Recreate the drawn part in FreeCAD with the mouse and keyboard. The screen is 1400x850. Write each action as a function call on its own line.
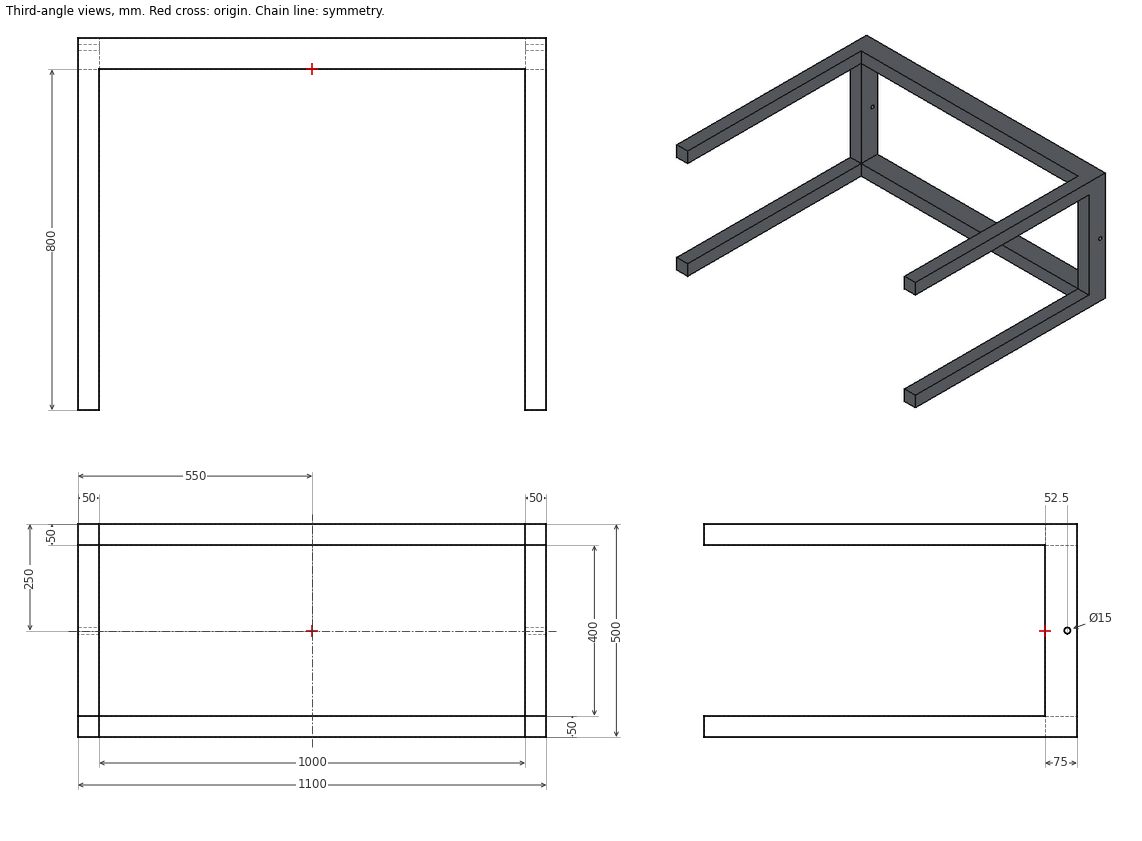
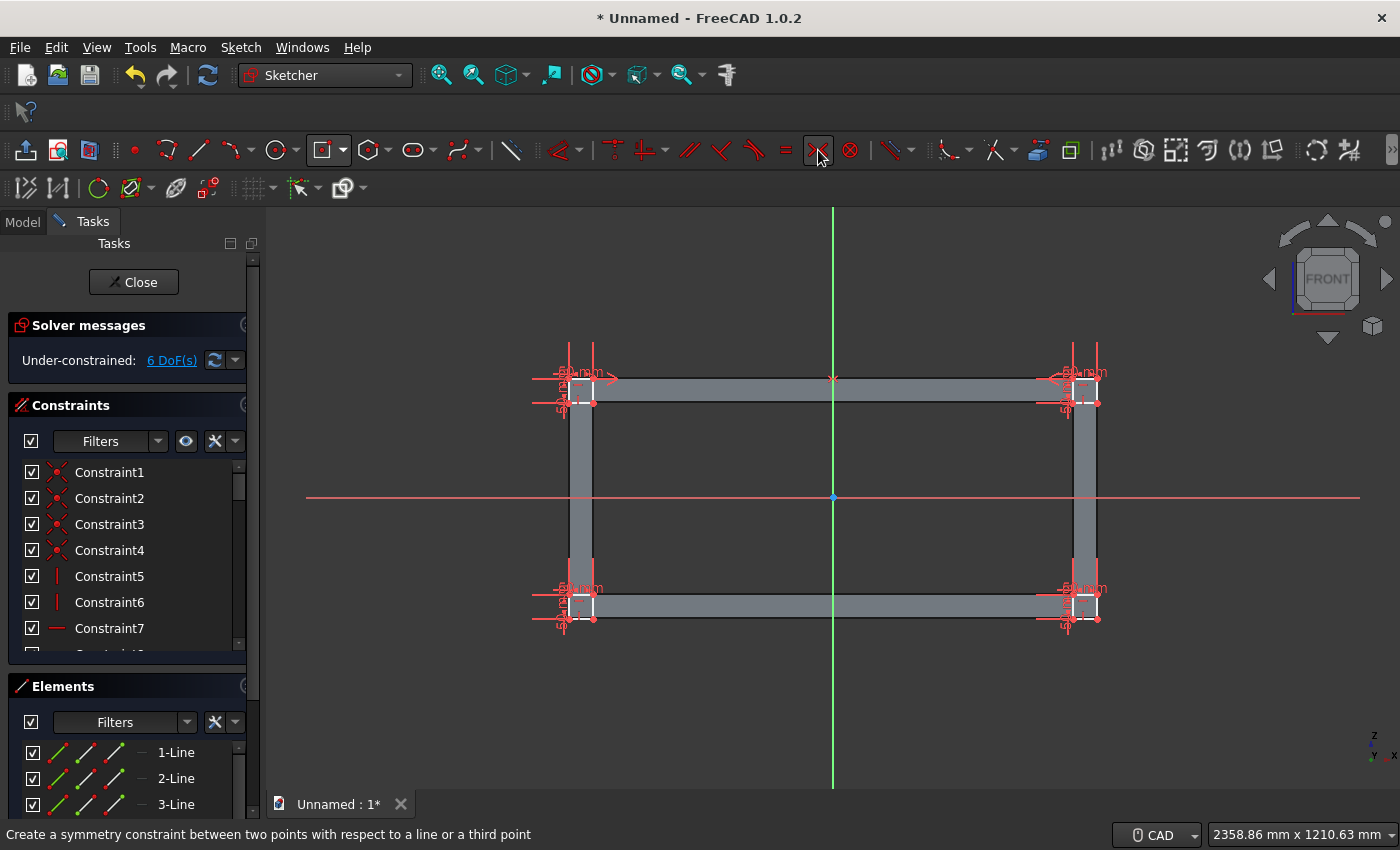
click(1073, 403)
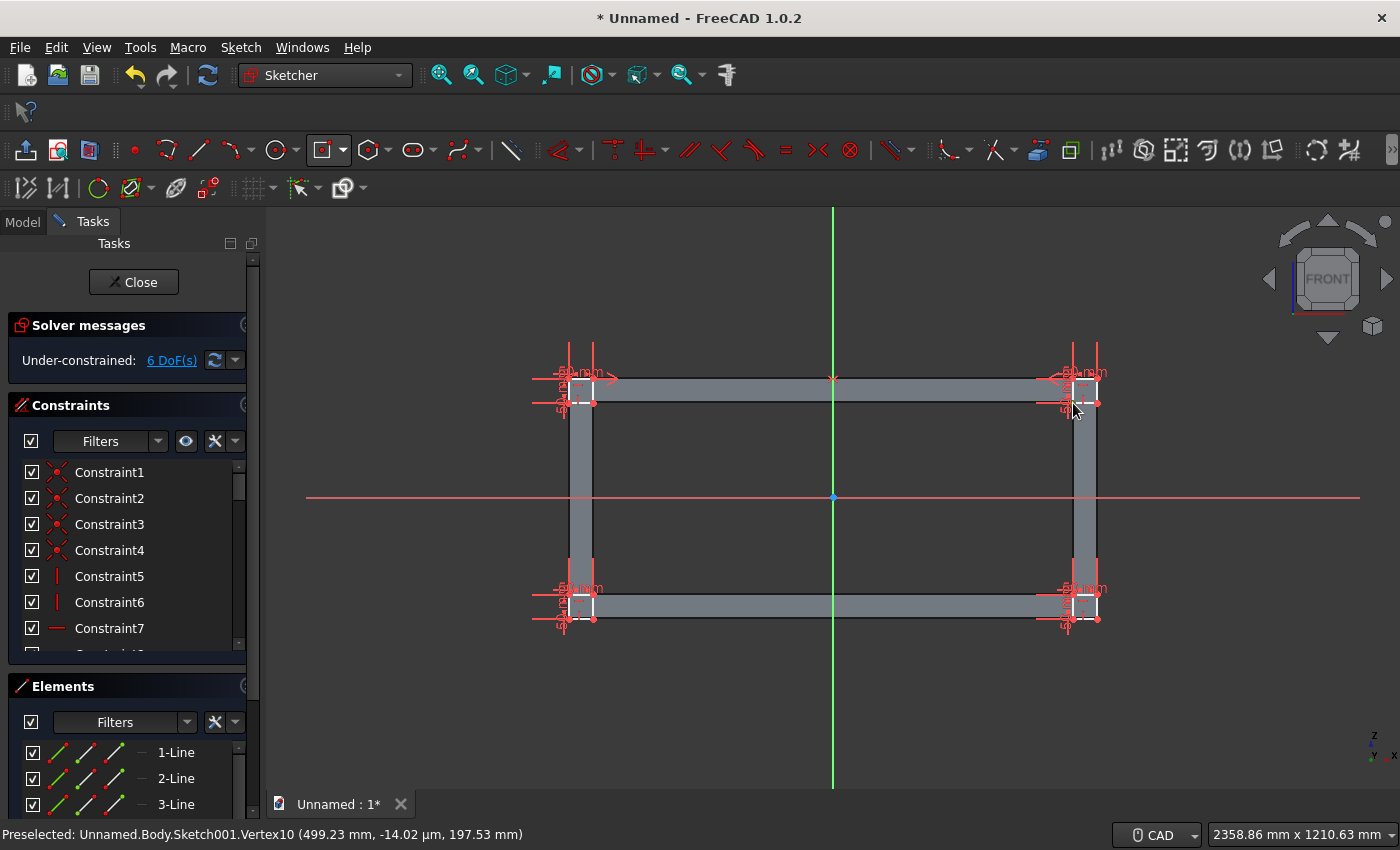
click(1073, 595)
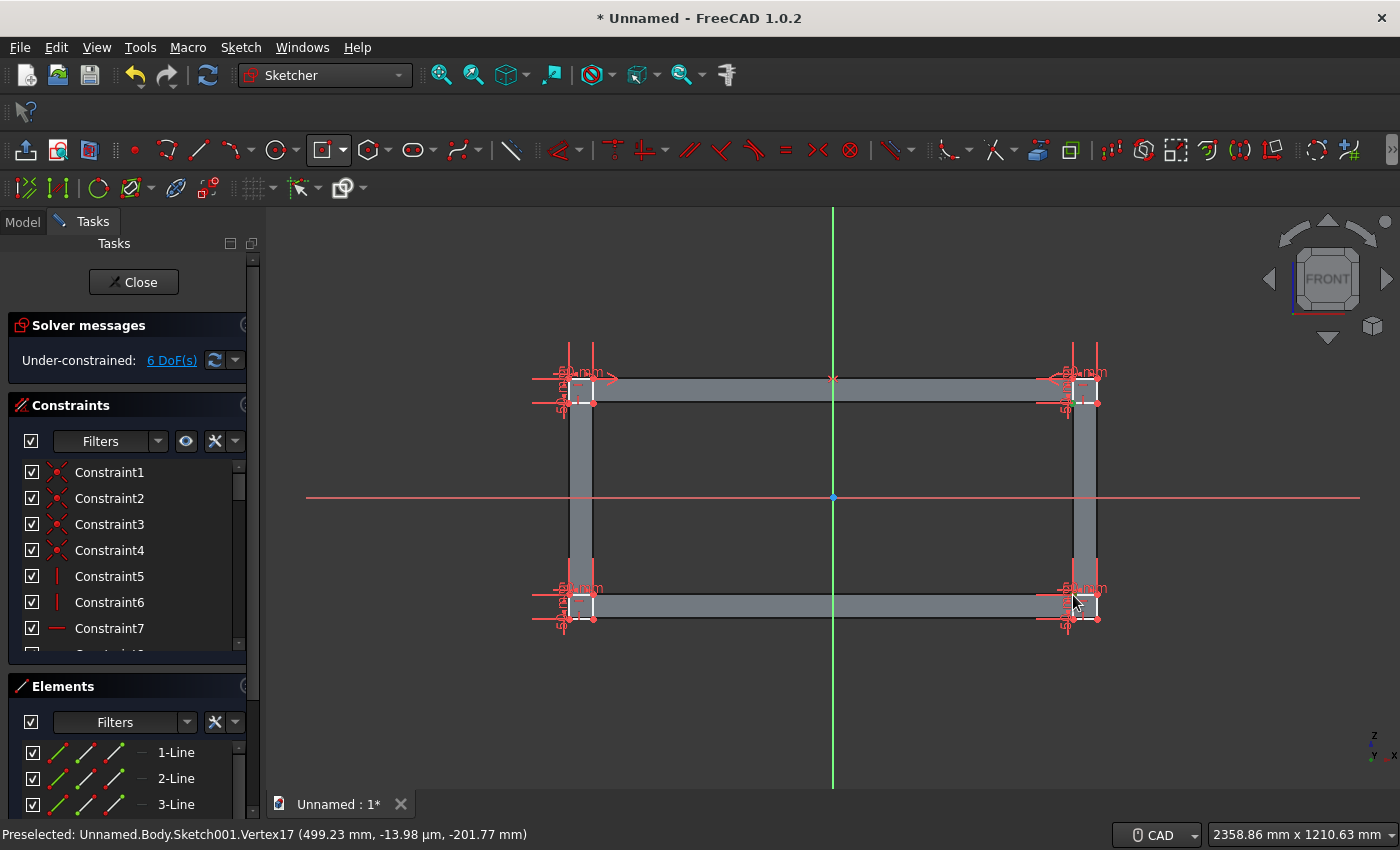
click(361, 498)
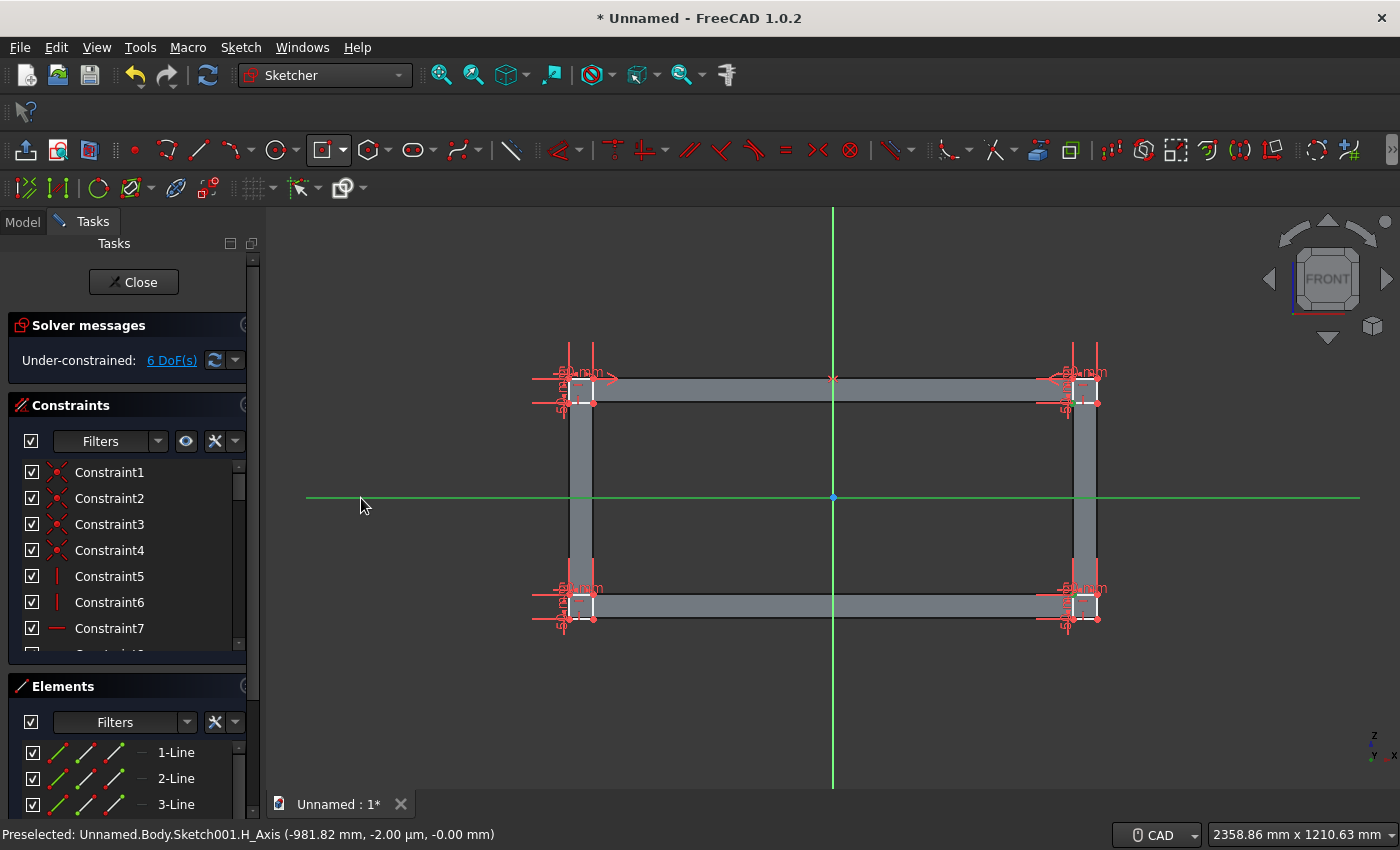
click(818, 150)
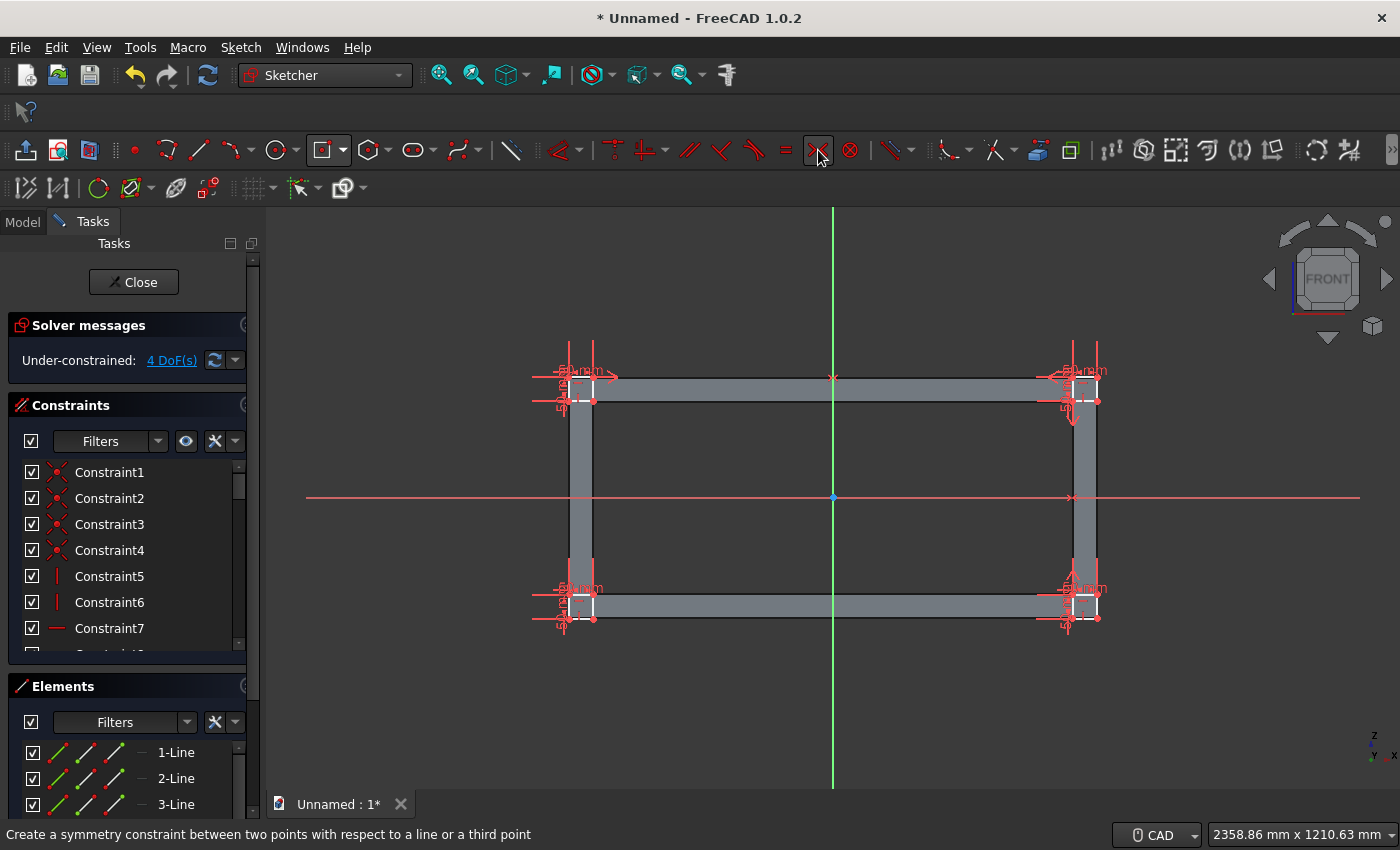
click(569, 401)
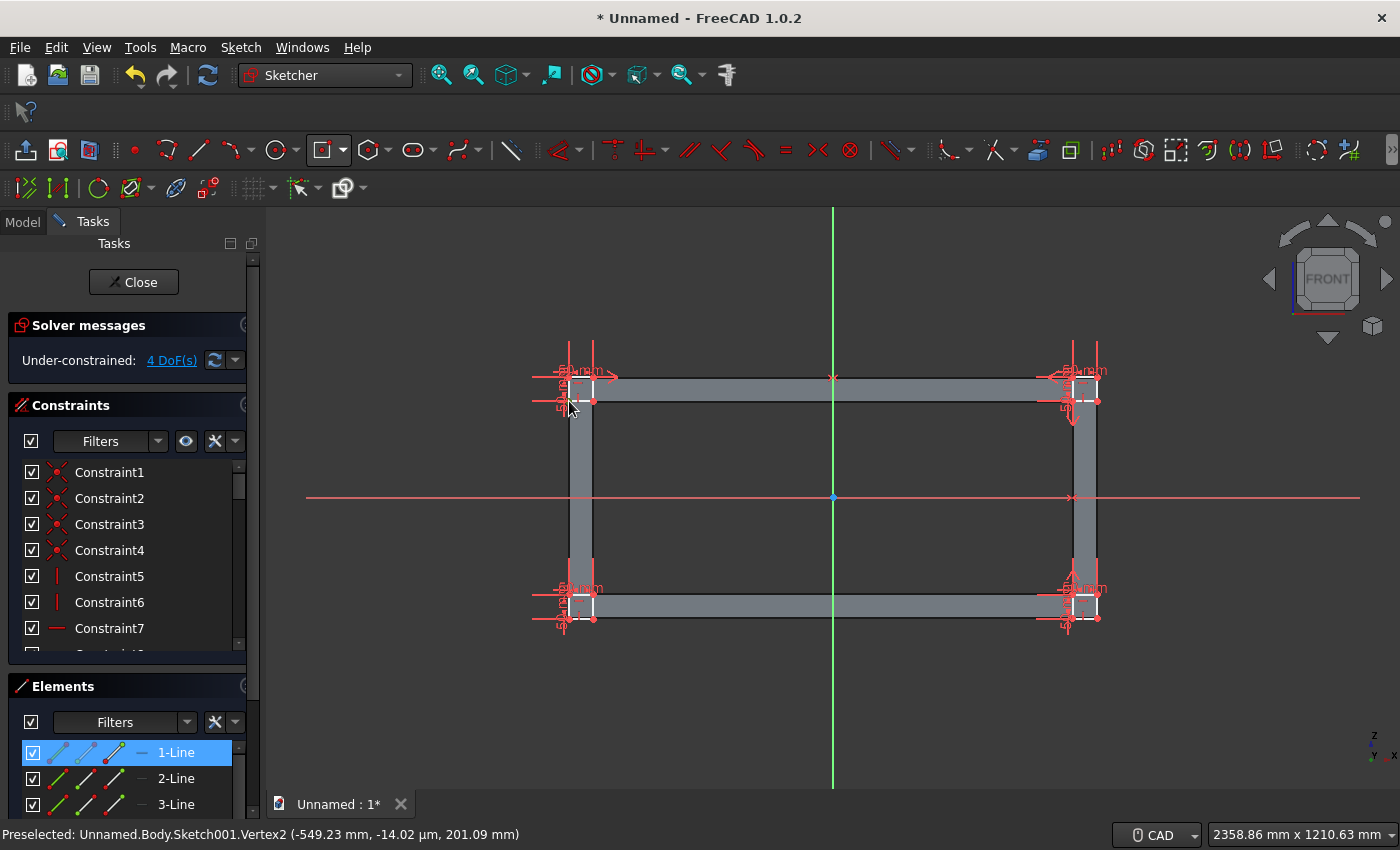
click(569, 595)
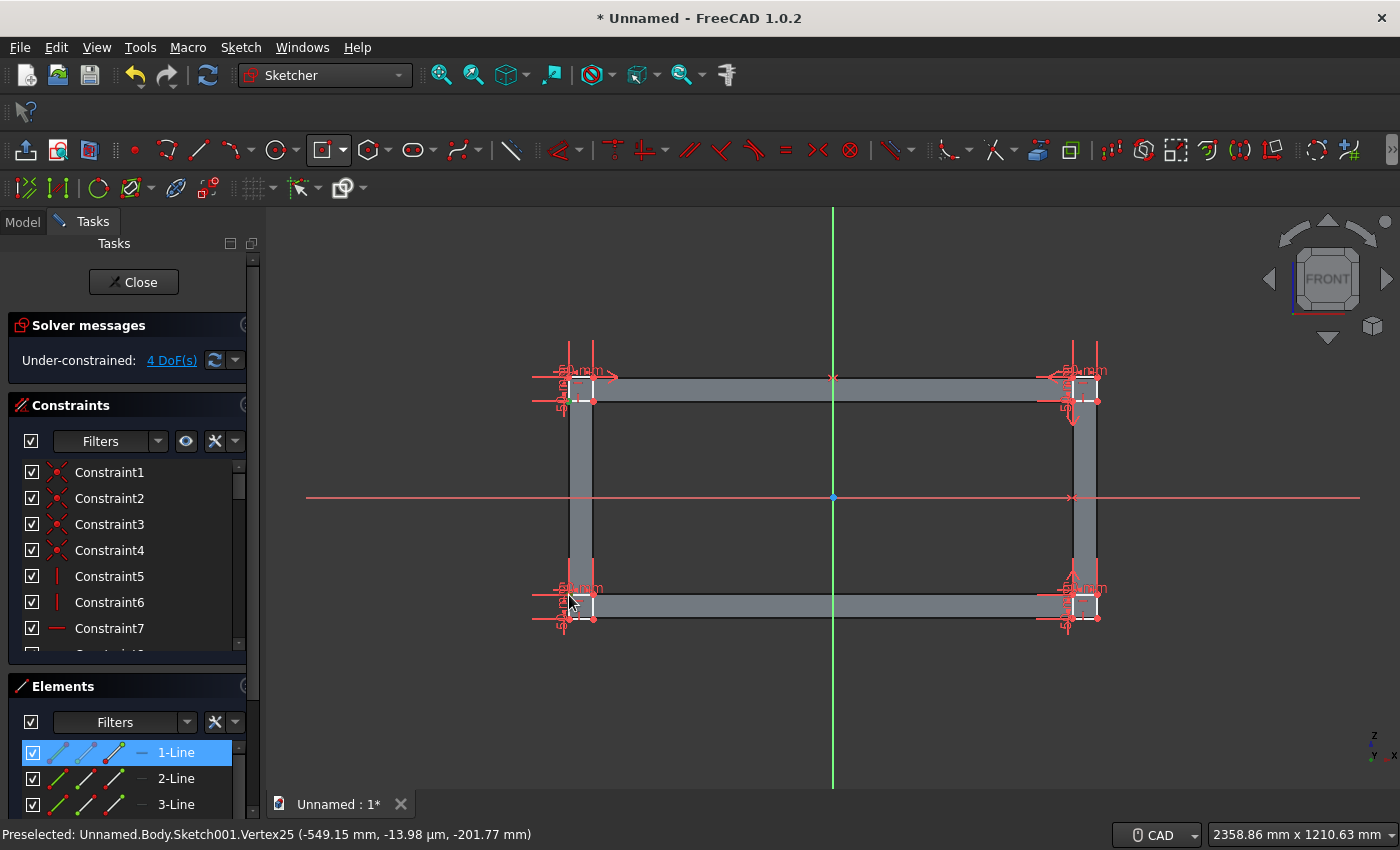
click(361, 498)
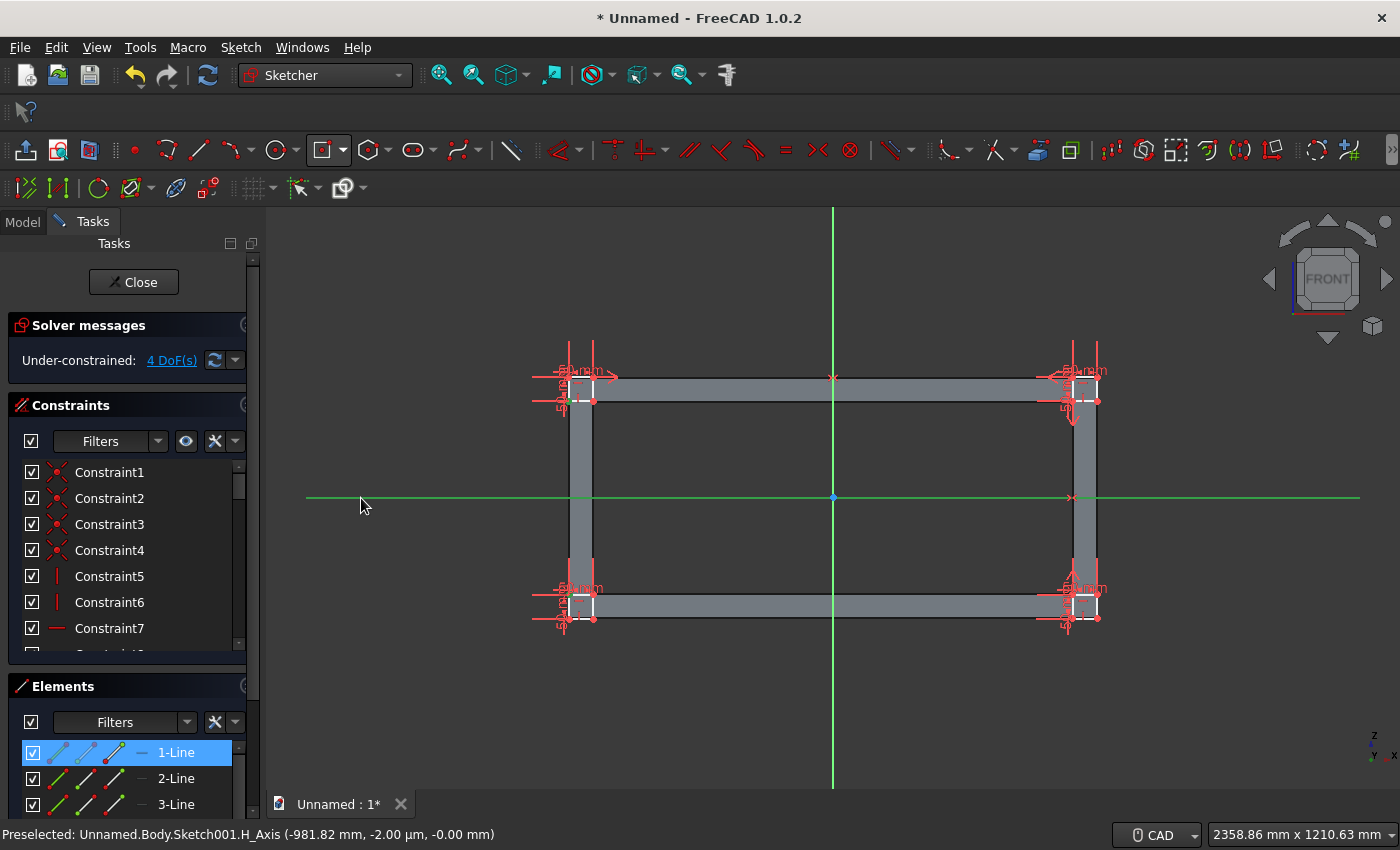
key(s)